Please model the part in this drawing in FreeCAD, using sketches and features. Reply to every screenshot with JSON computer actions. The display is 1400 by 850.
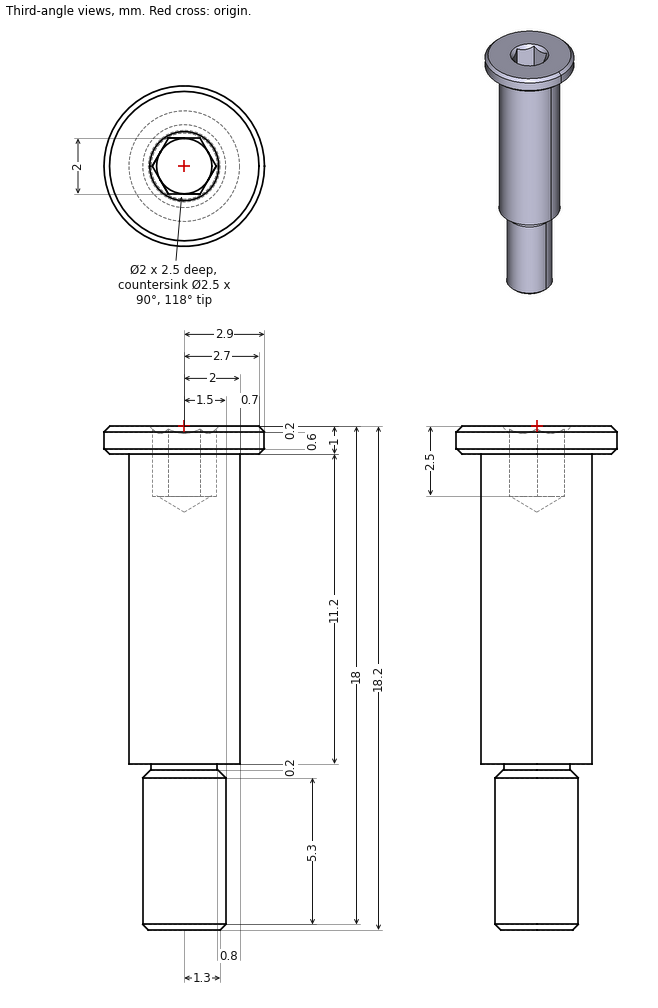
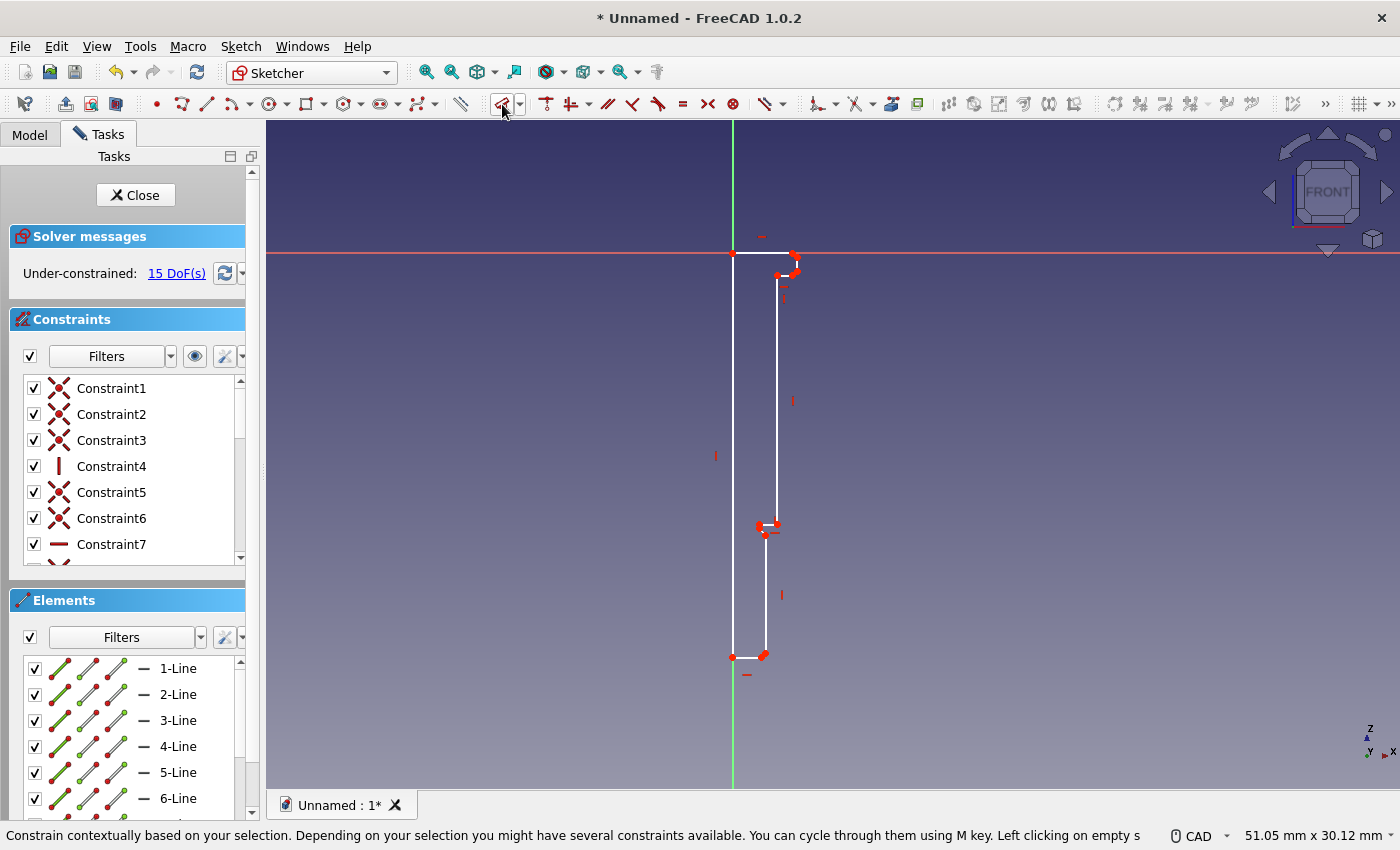
{"action": "scroll", "coordinate": [793, 276], "scroll_direction": "up", "scroll_amount": 4}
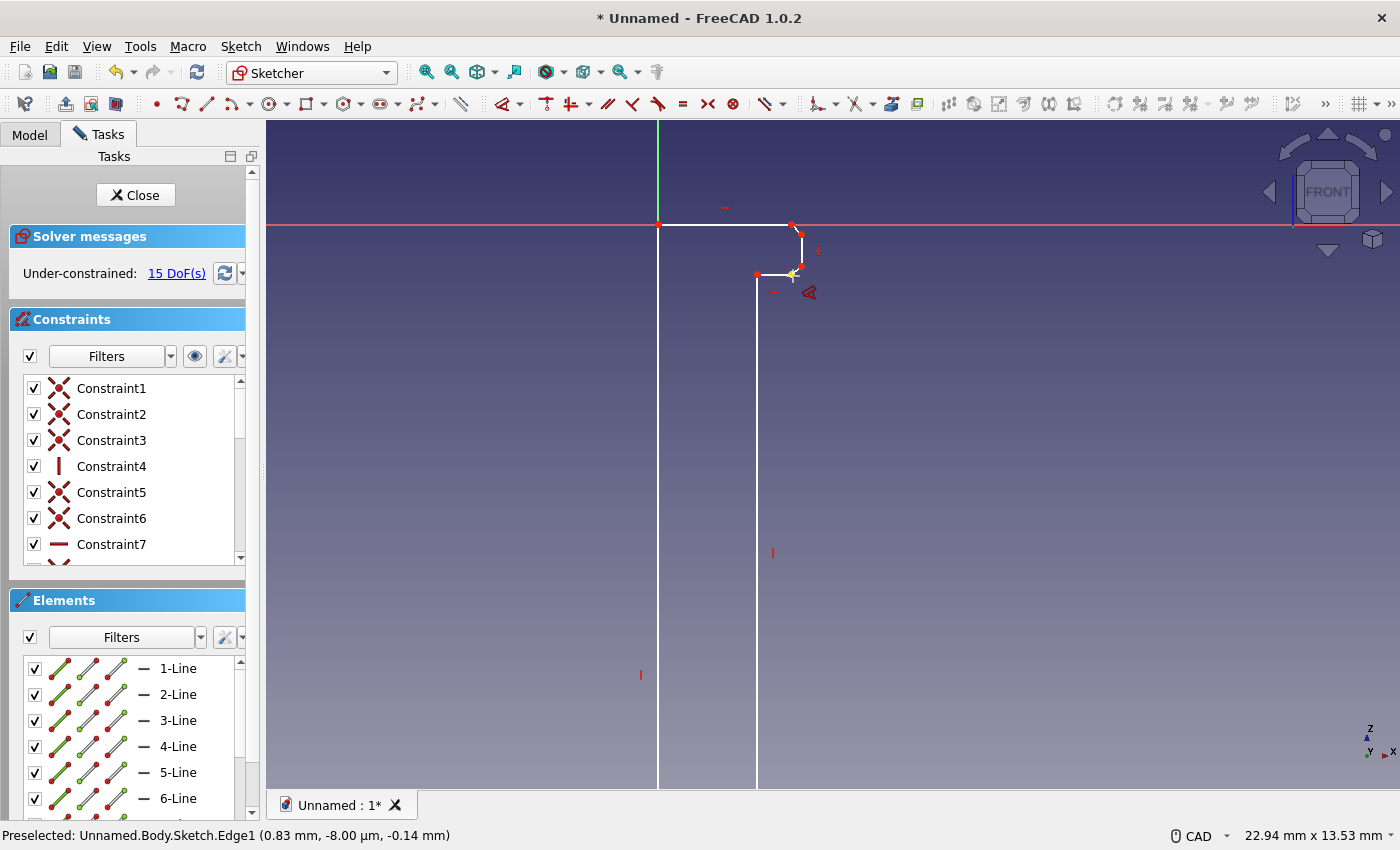
{"action": "left_click", "coordinate": [791, 275]}
{"action": "left_click", "coordinate": [624, 250]}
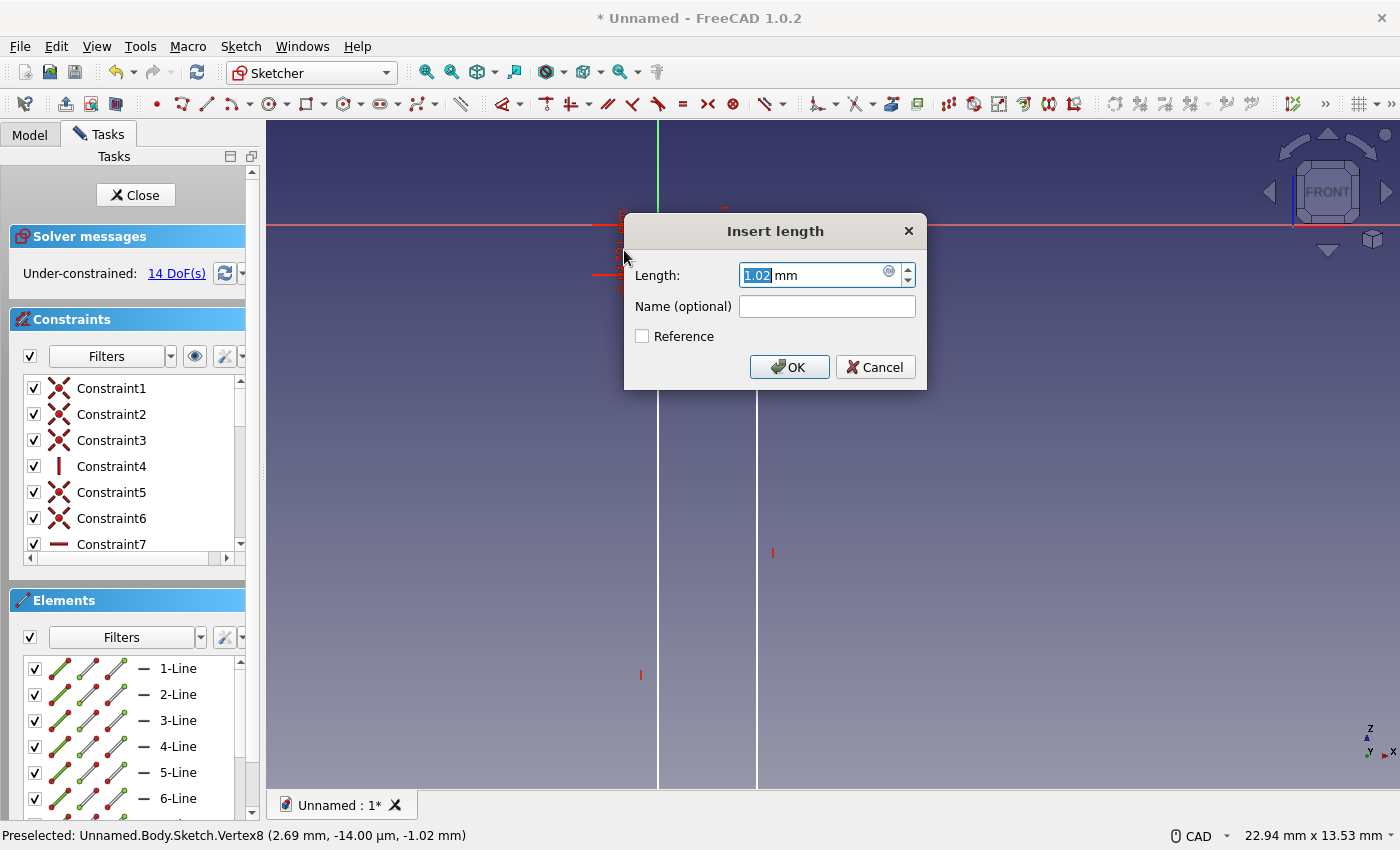
{"action": "type", "text": "1"}
{"action": "key", "text": "Return"}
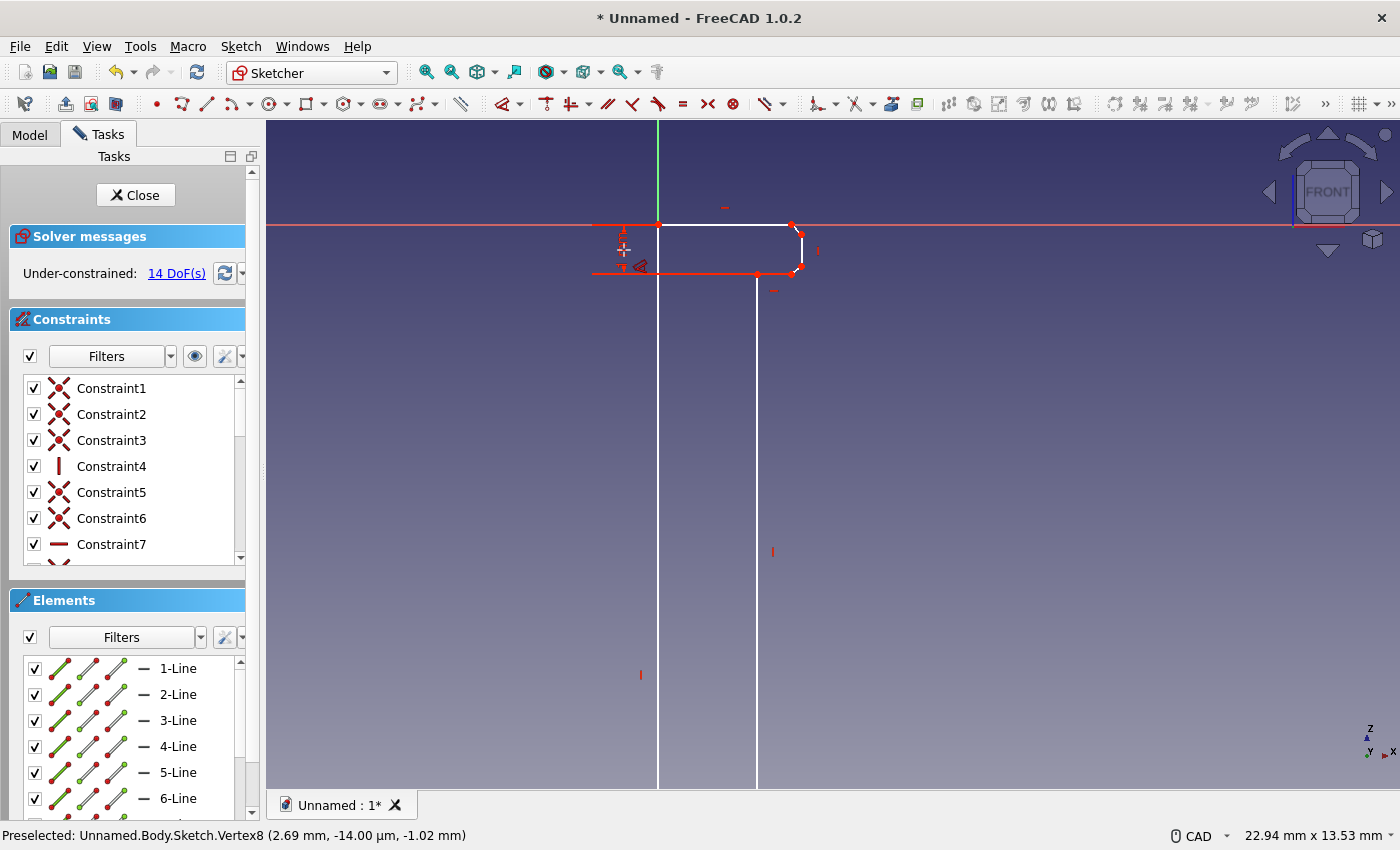
{"action": "left_click", "coordinate": [757, 274]}
{"action": "left_click", "coordinate": [708, 191]}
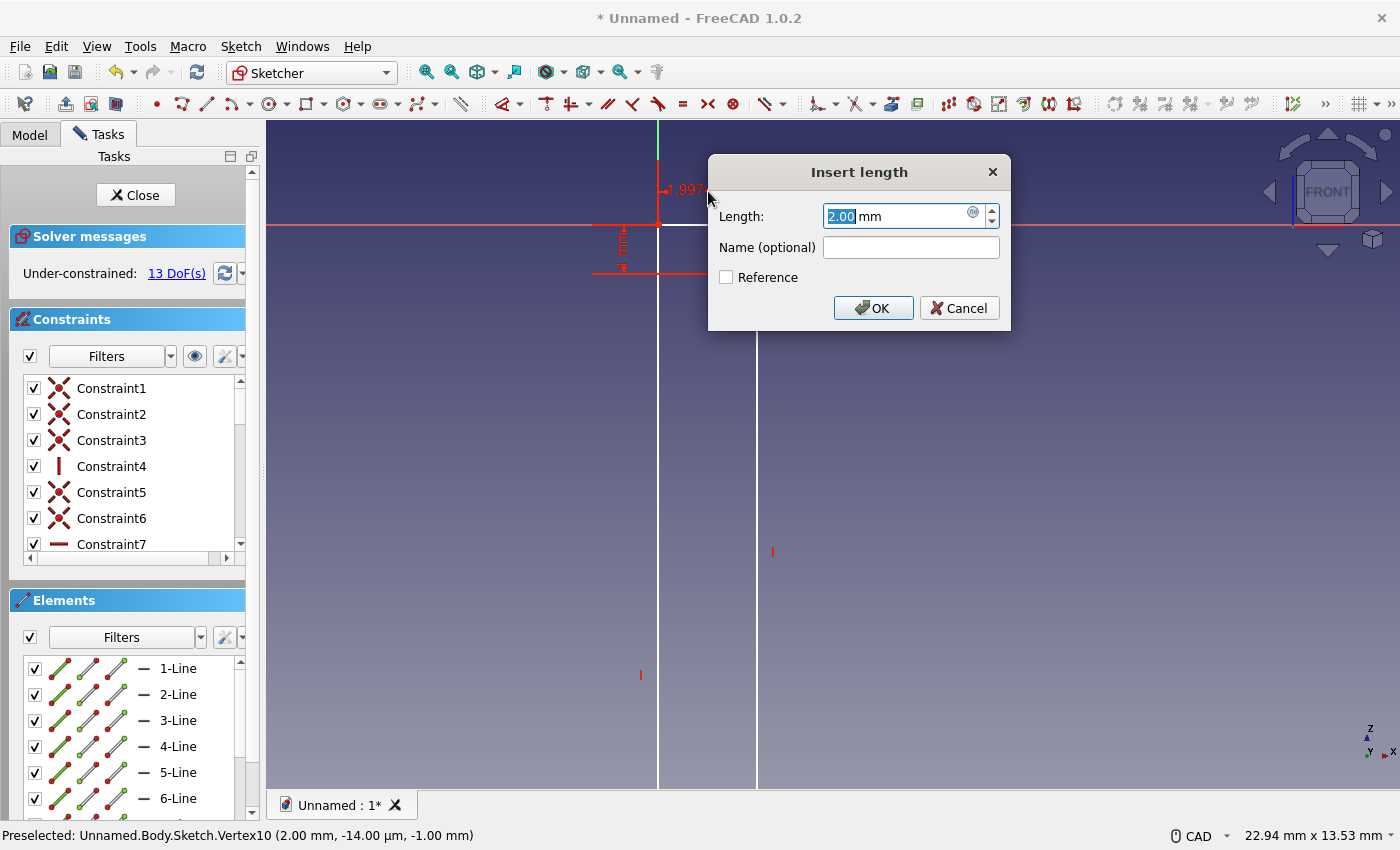
{"action": "type", "text": "2"}
{"action": "key", "text": "Return"}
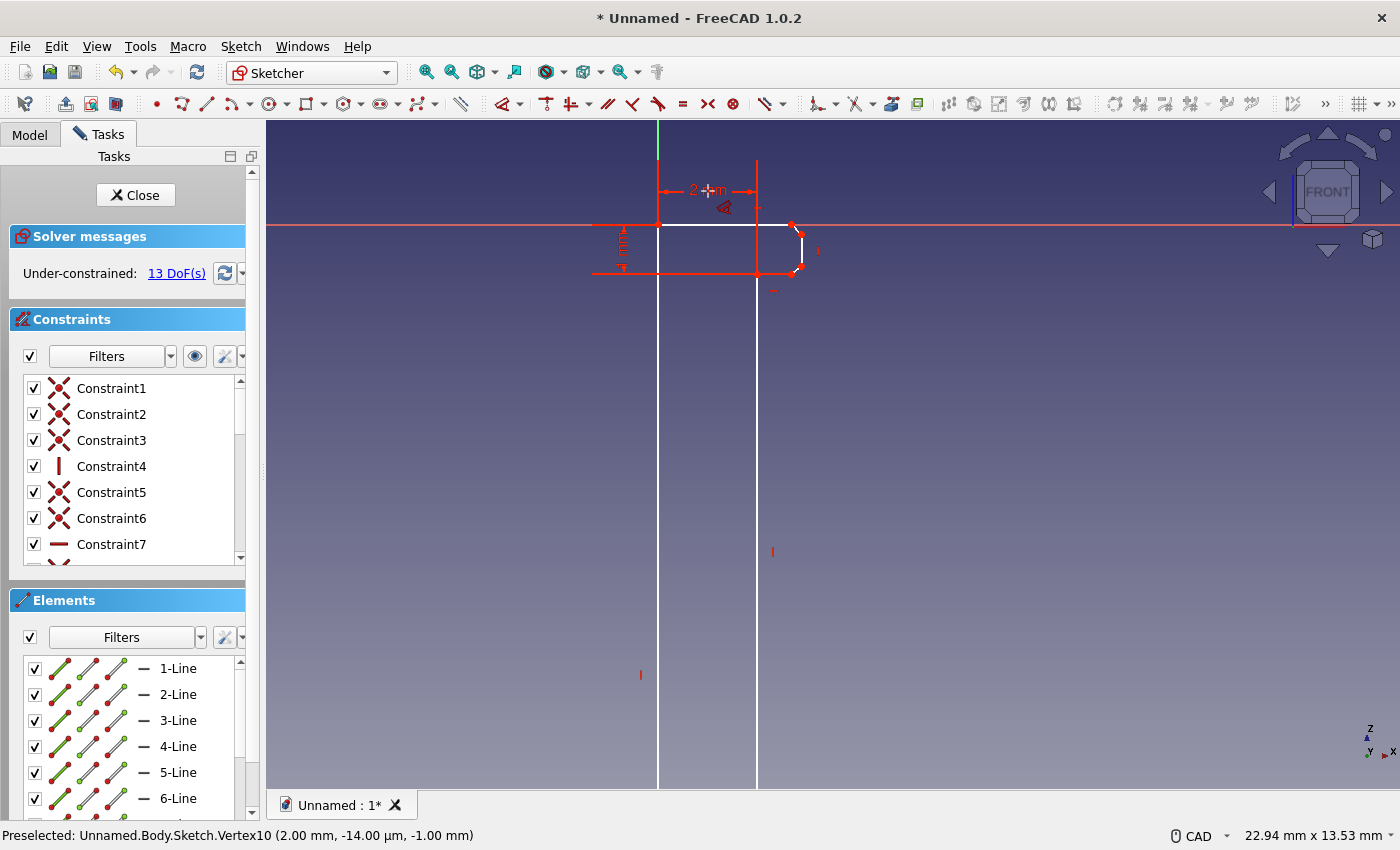
{"action": "left_click", "coordinate": [698, 225]}
{"action": "left_click", "coordinate": [725, 259]}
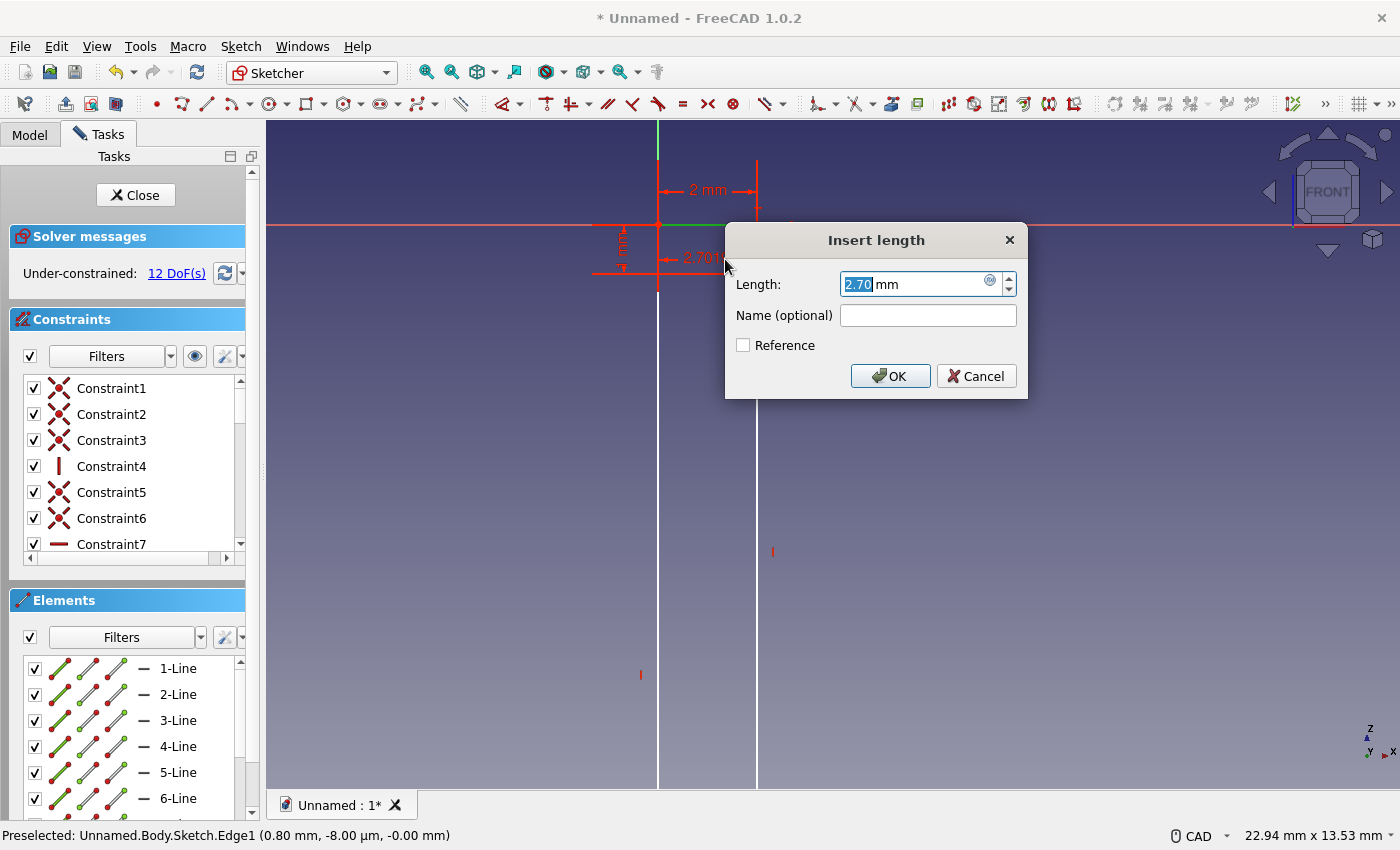
{"action": "type", "text": "2.7"}
{"action": "key", "text": "Return"}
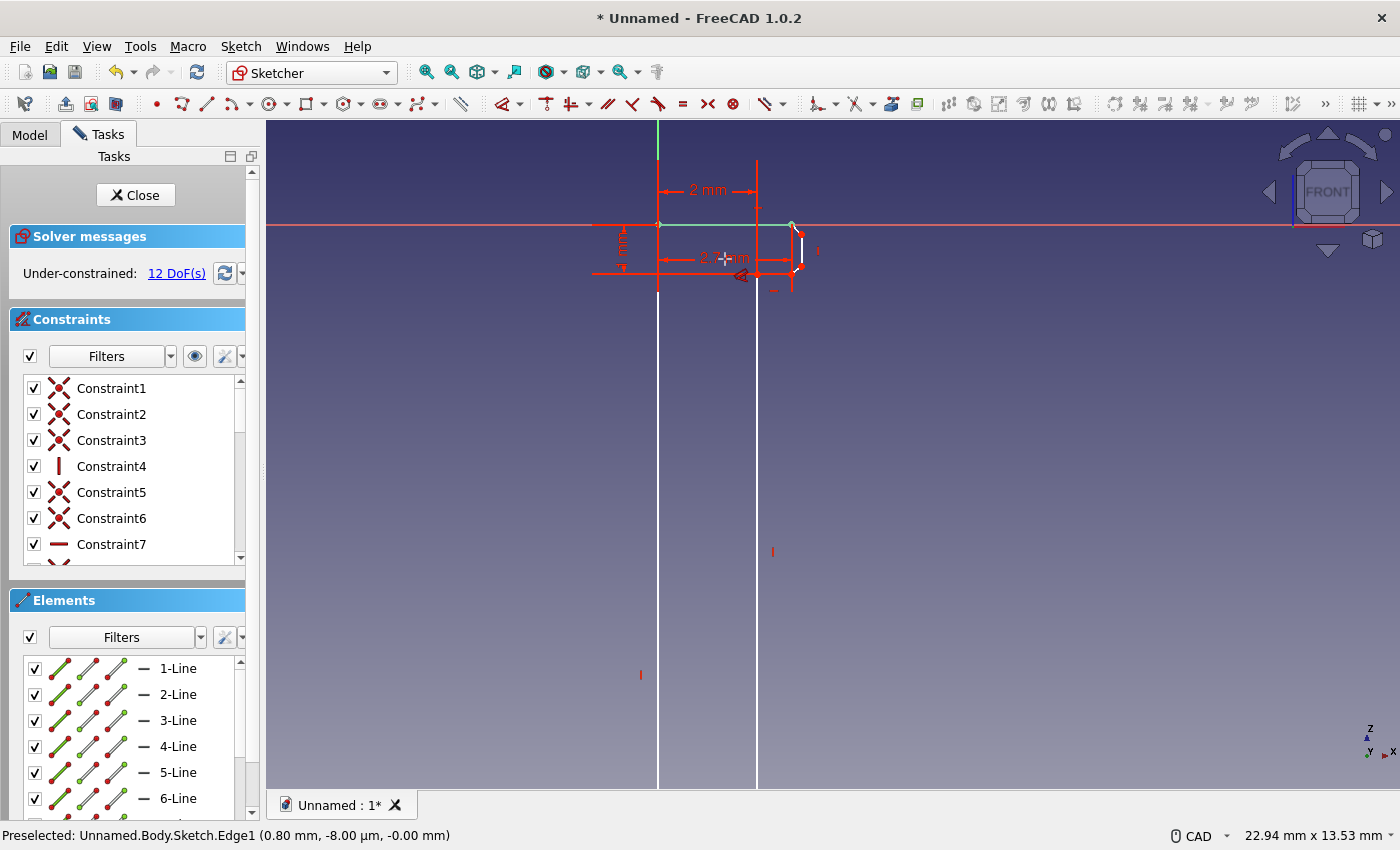
{"action": "scroll", "coordinate": [802, 244], "scroll_direction": "up", "scroll_amount": 2}